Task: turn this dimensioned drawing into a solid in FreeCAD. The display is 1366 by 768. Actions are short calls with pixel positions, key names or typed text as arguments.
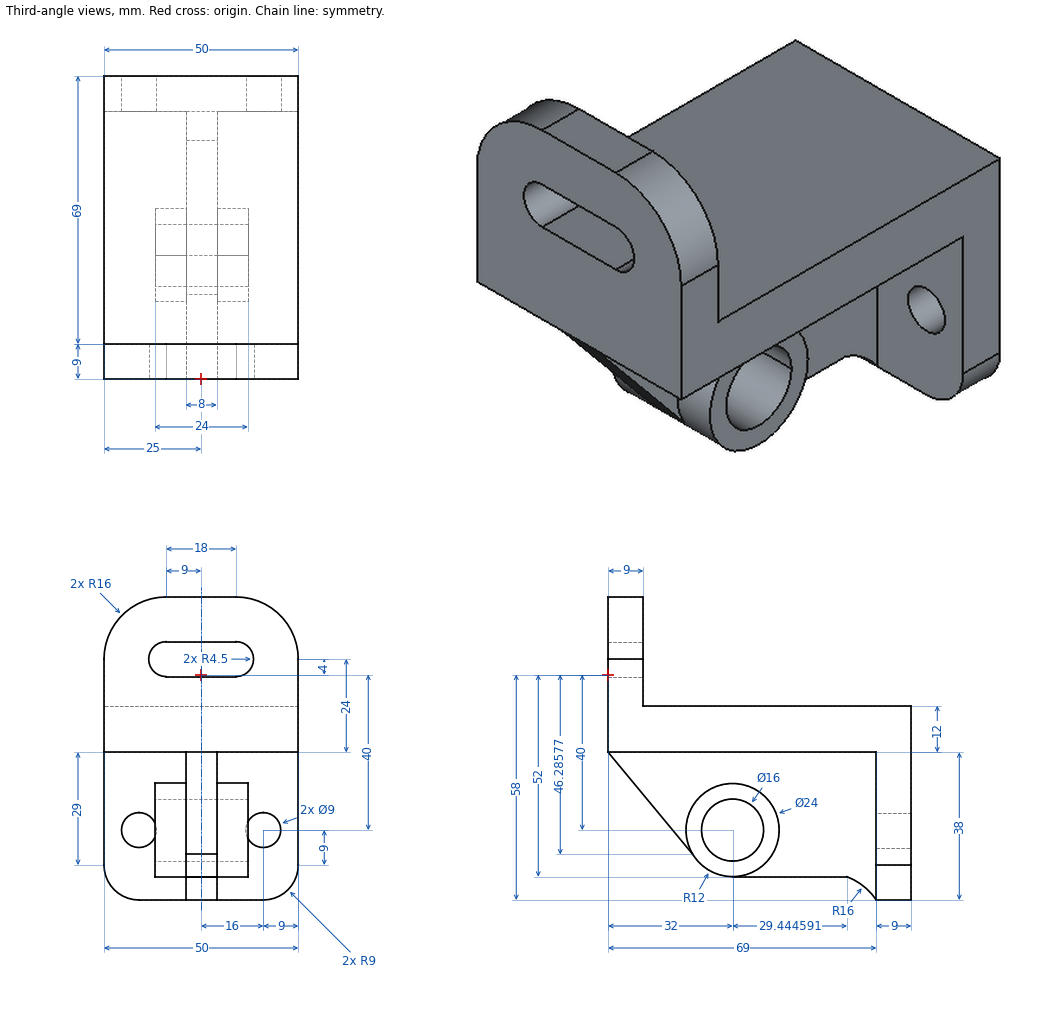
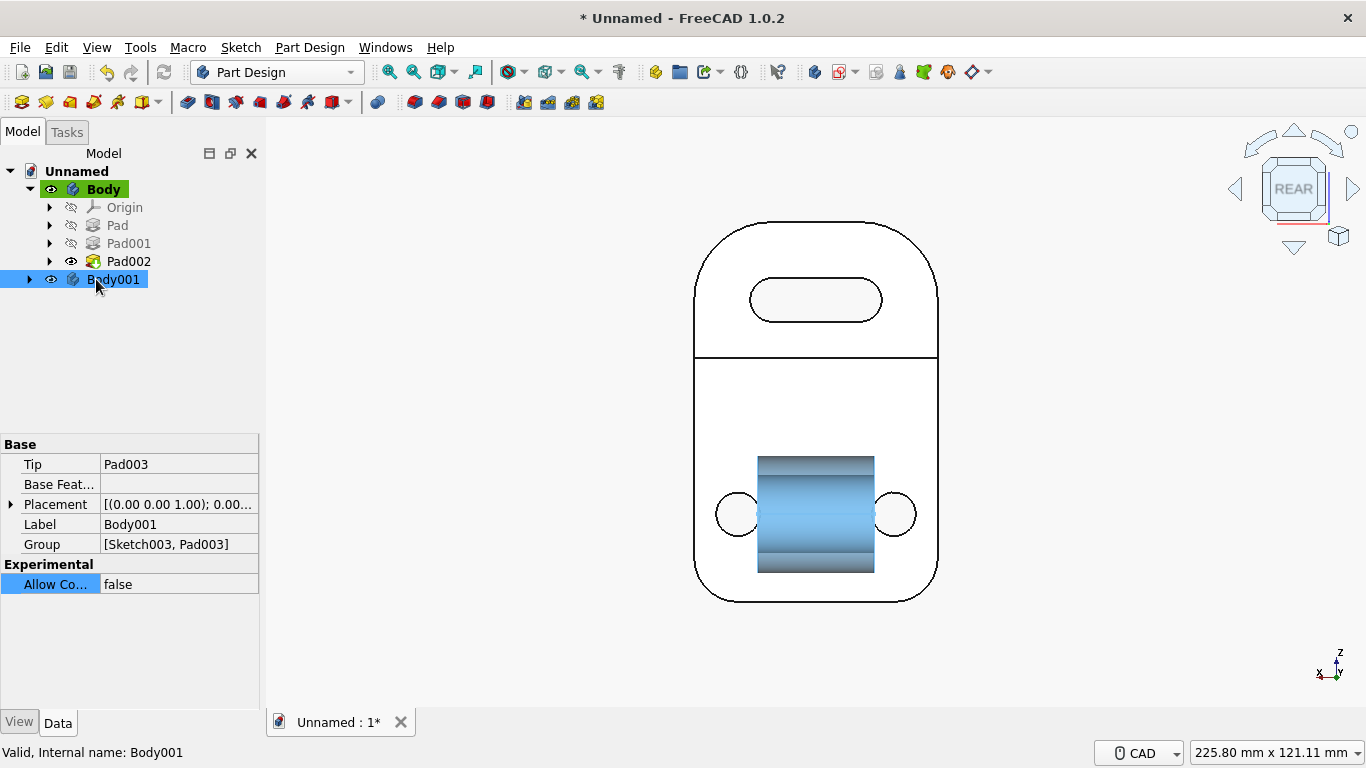
click(378, 102)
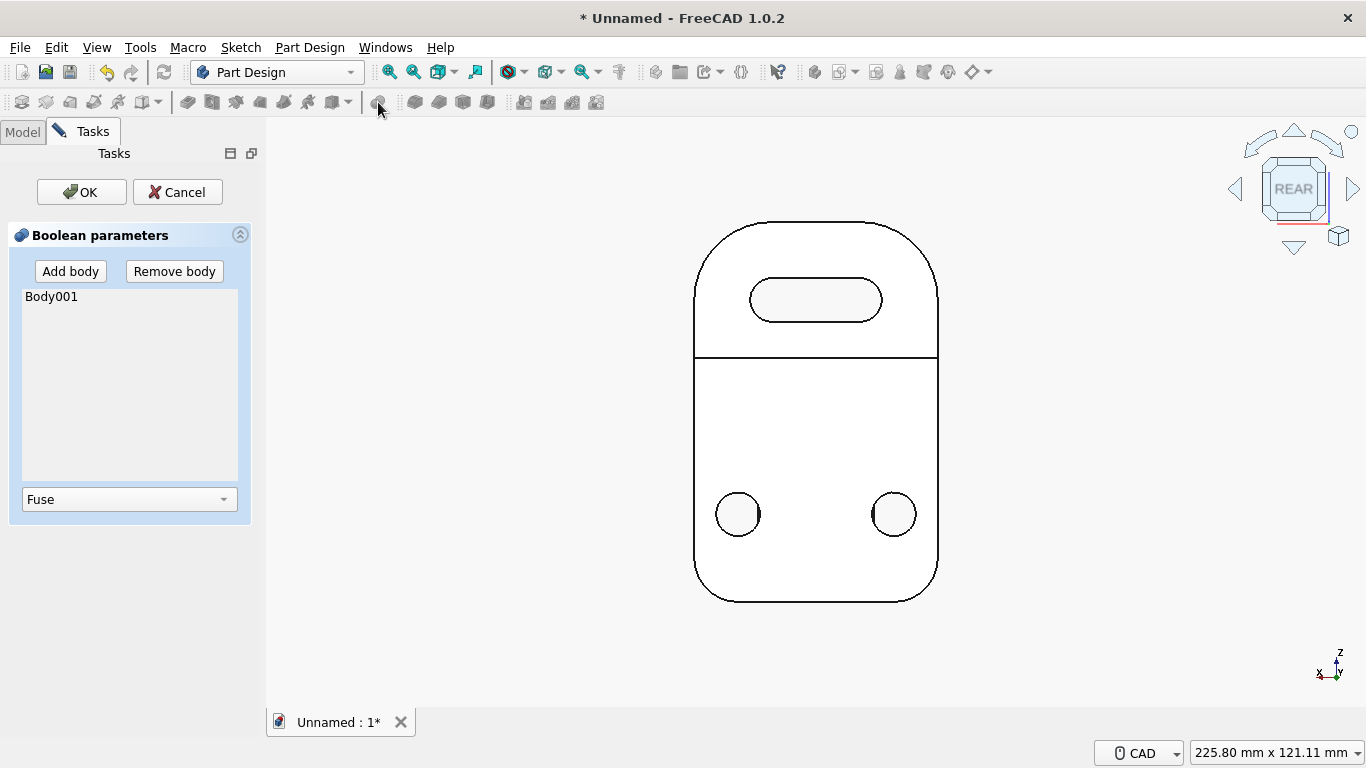
click(82, 192)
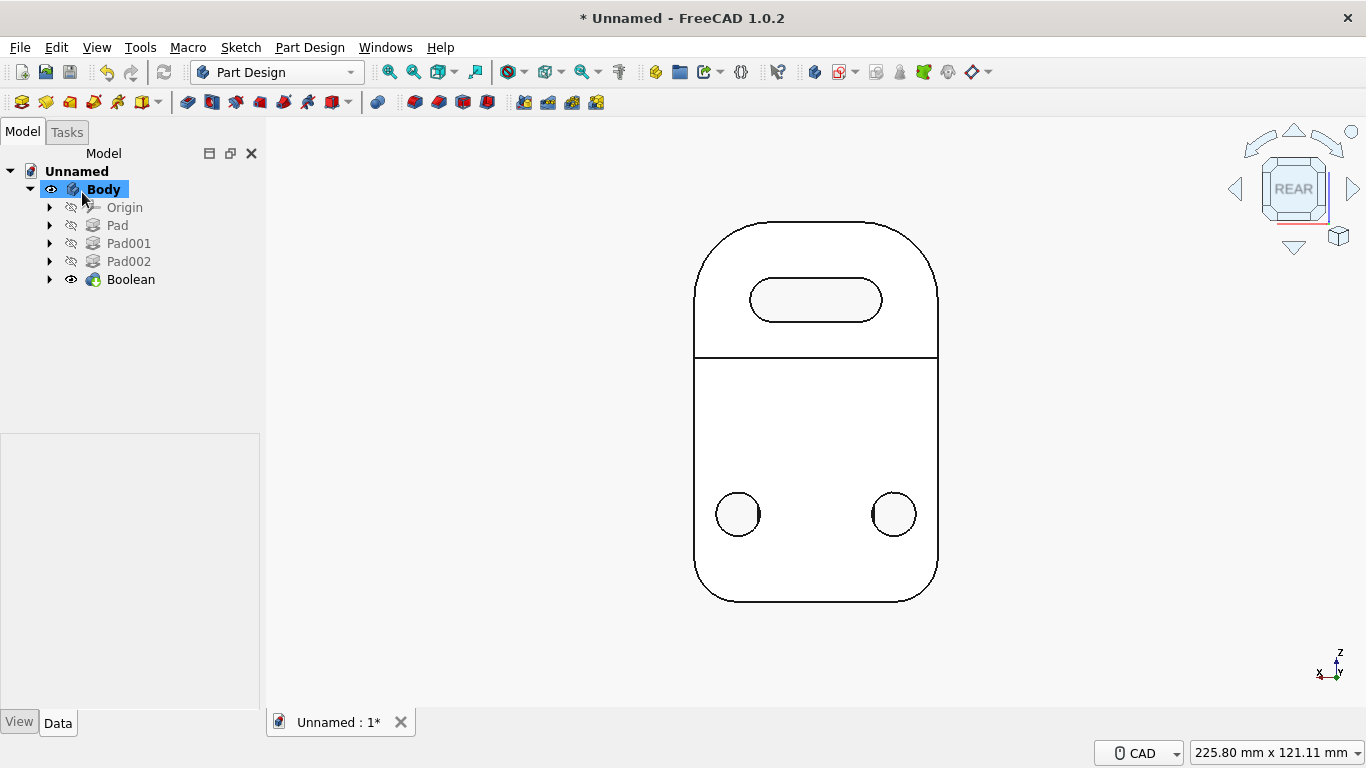
click(840, 72)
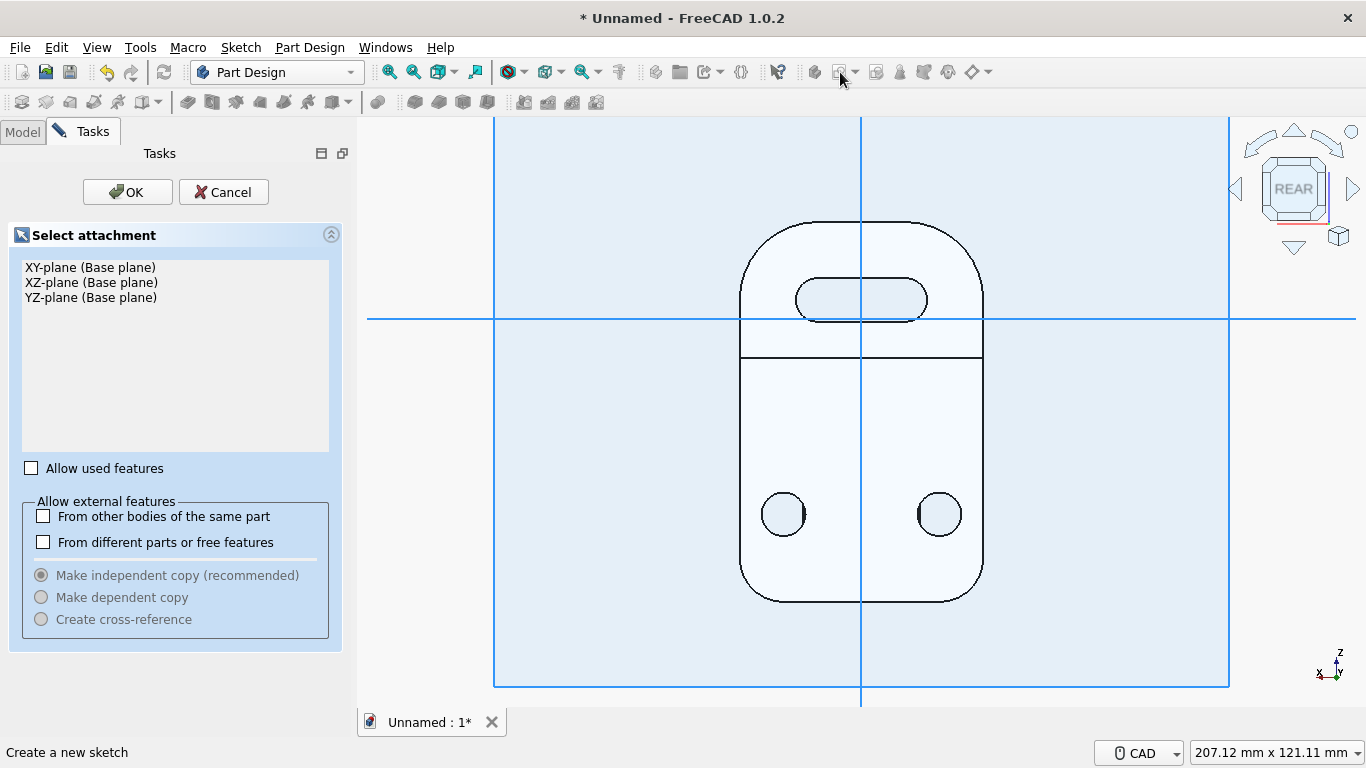
click(82, 298)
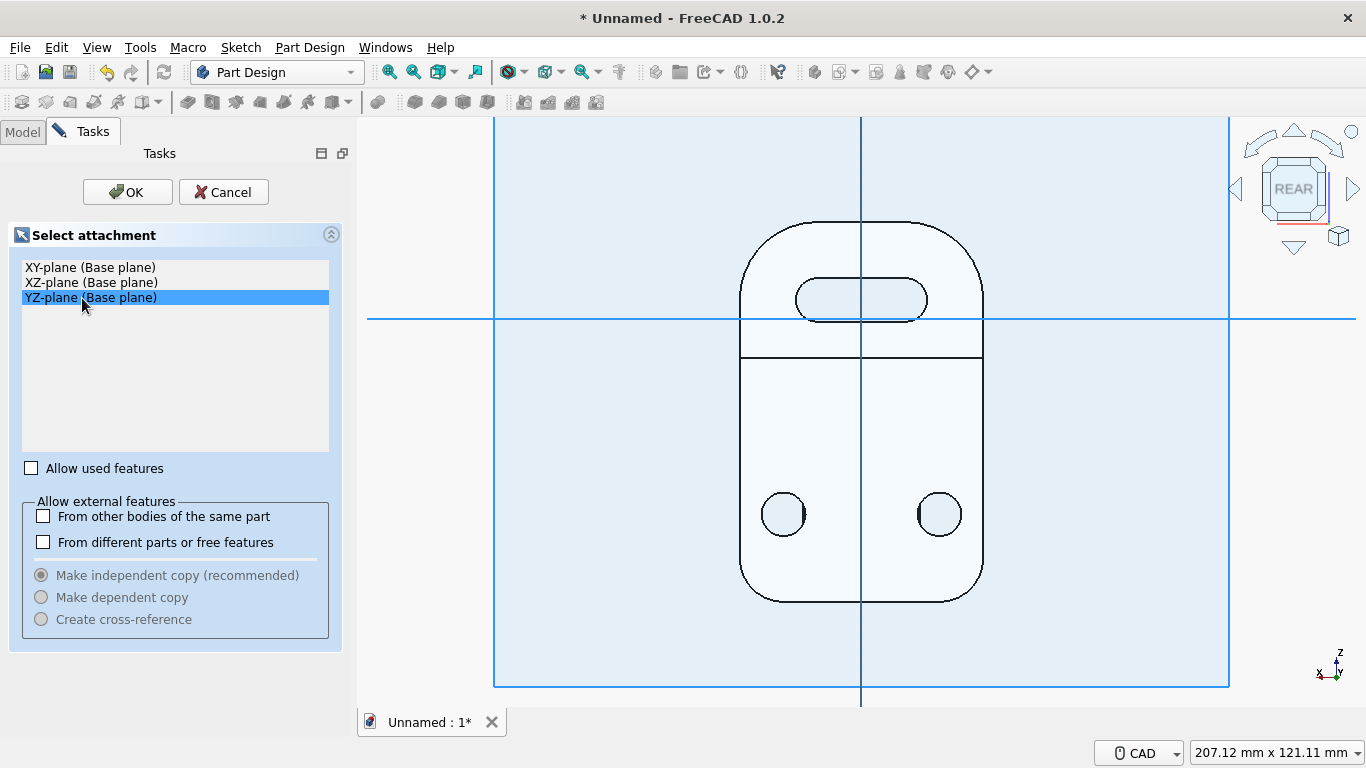
click(128, 192)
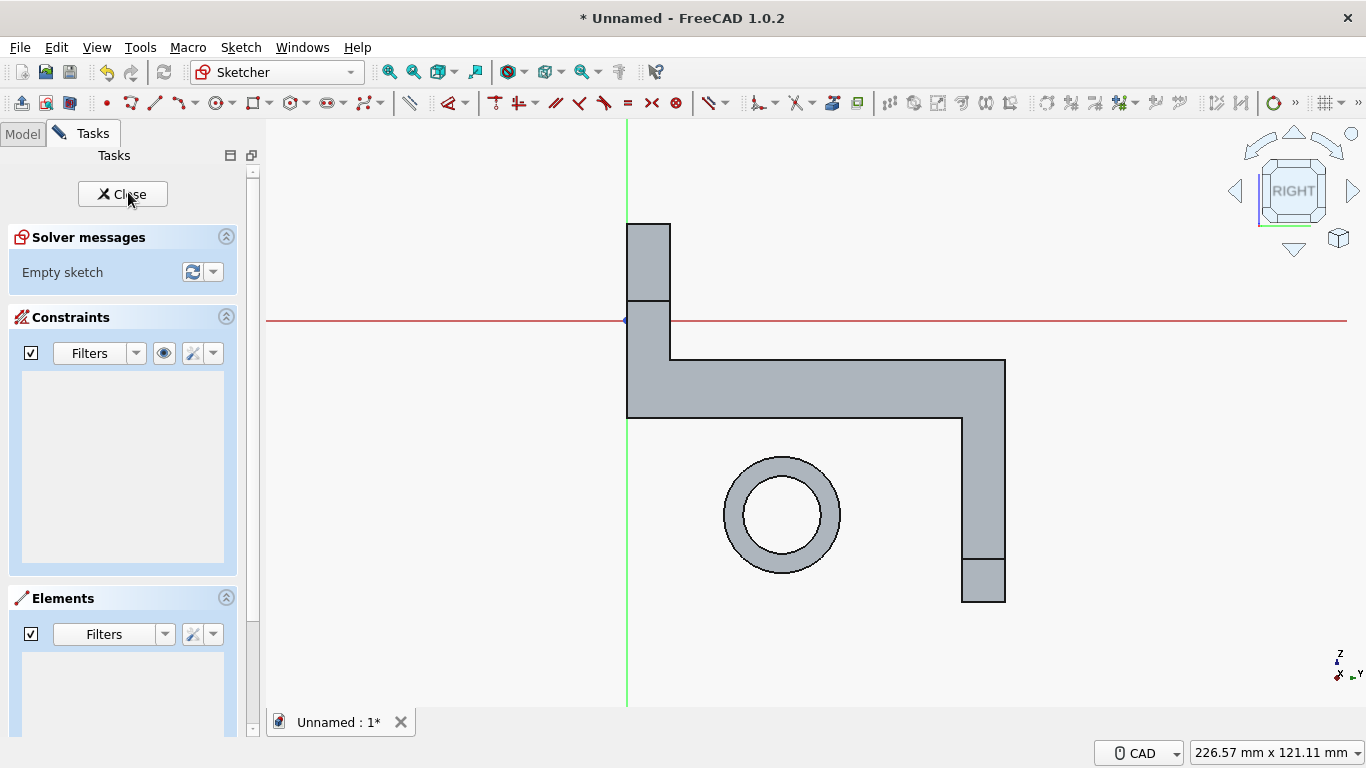
click(70, 104)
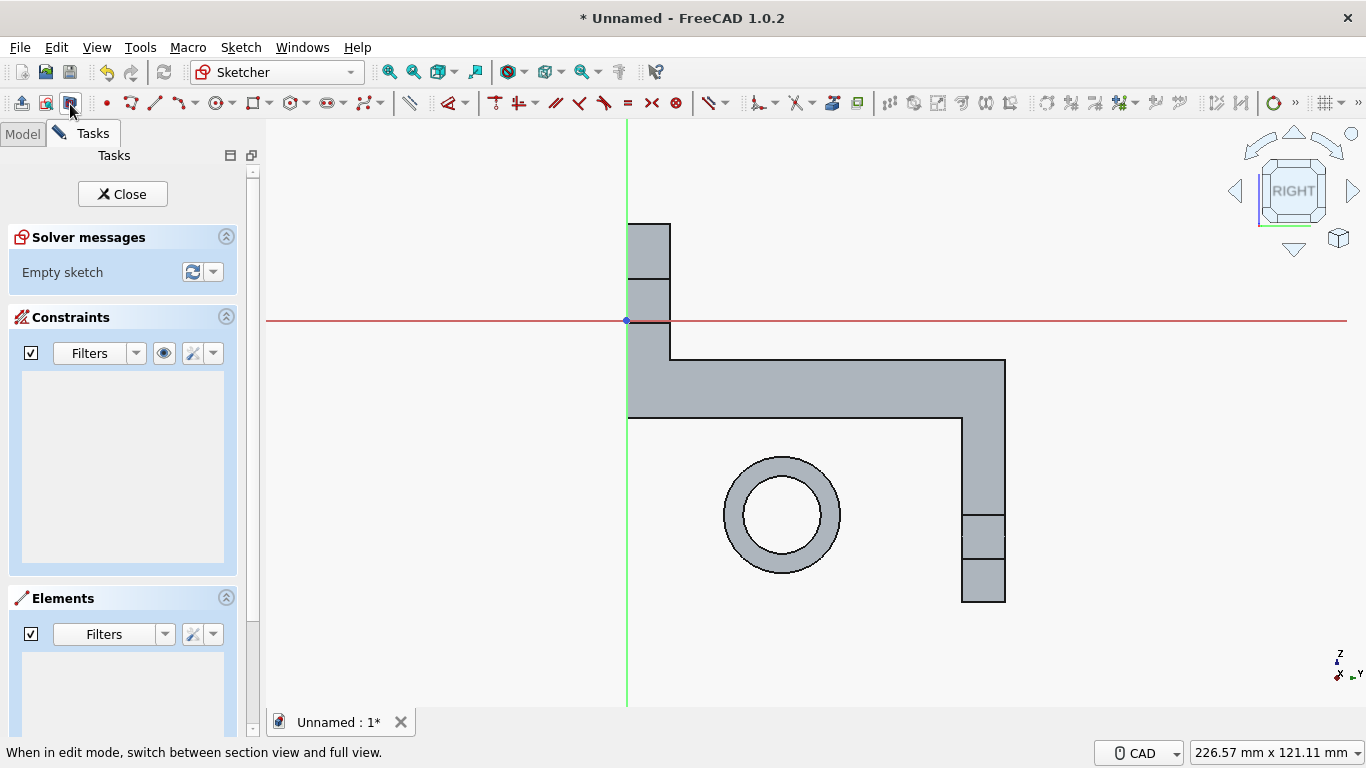
click(156, 104)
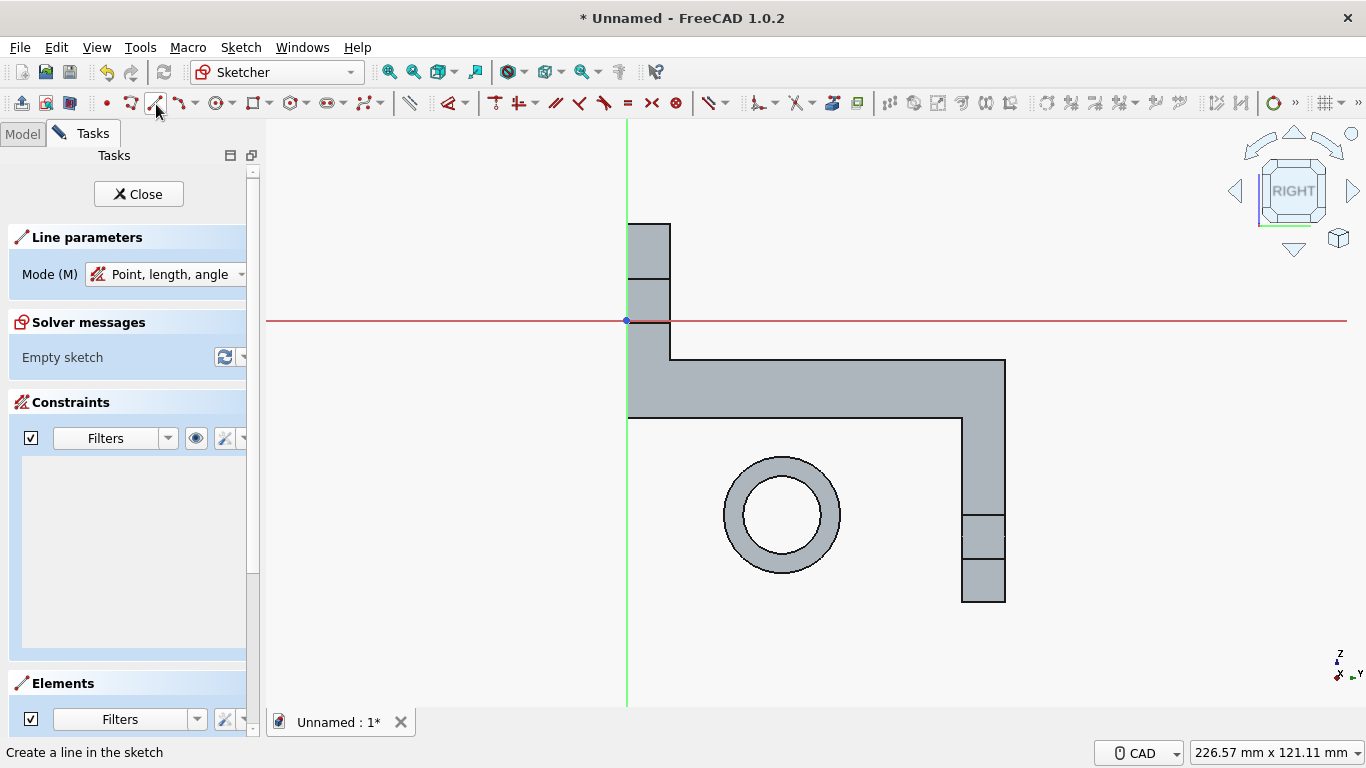
click(782, 573)
click(925, 573)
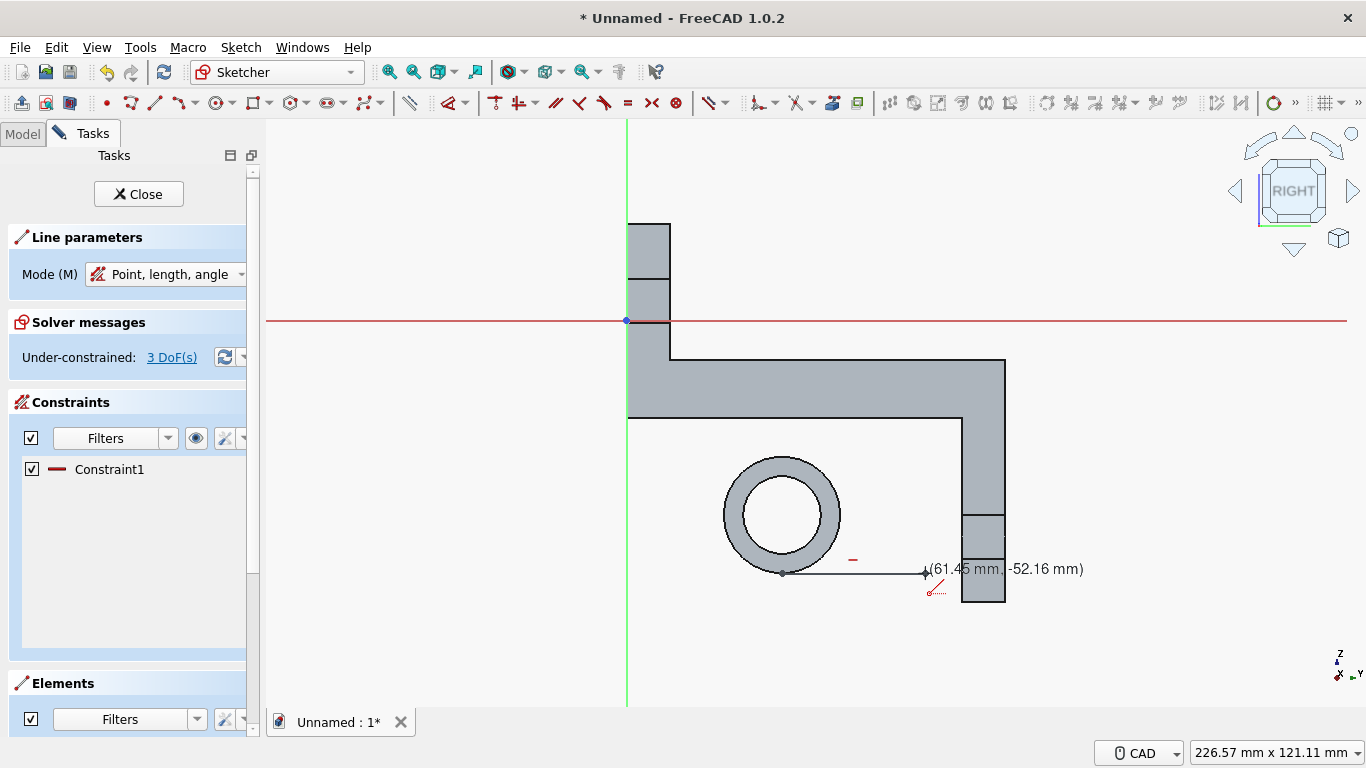
click(132, 104)